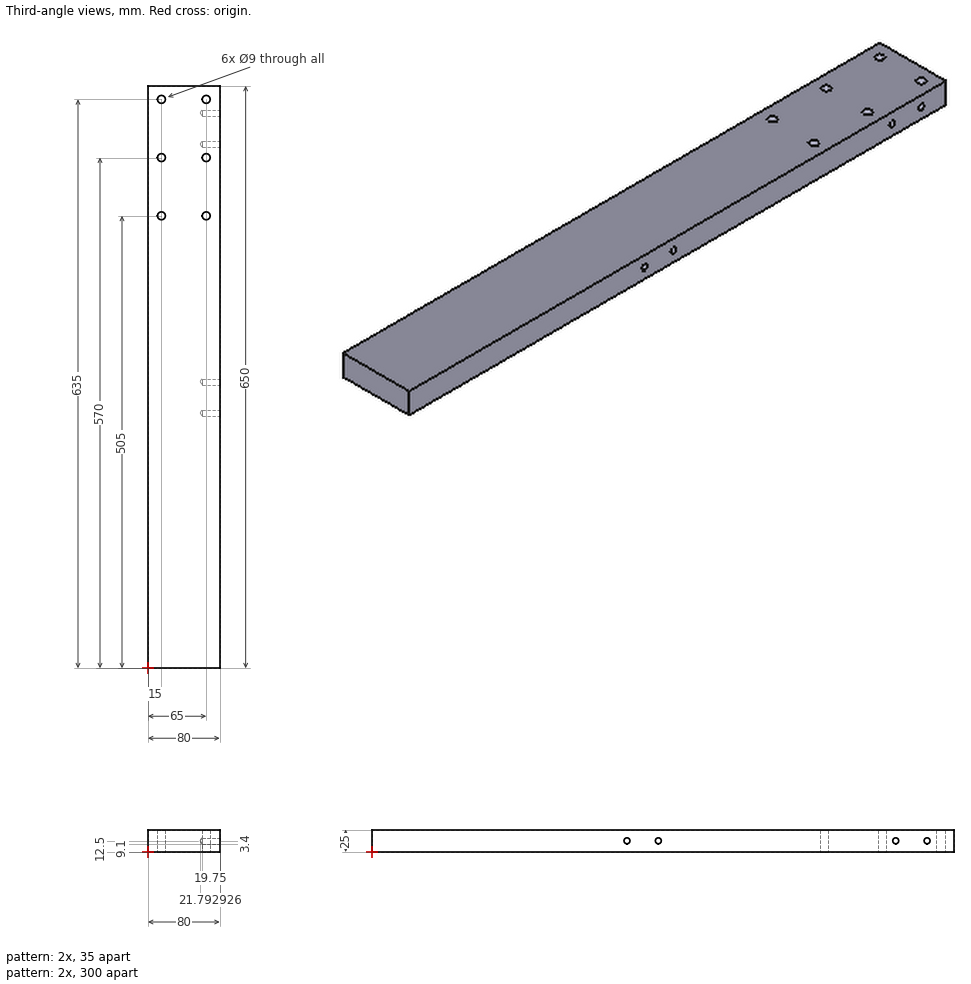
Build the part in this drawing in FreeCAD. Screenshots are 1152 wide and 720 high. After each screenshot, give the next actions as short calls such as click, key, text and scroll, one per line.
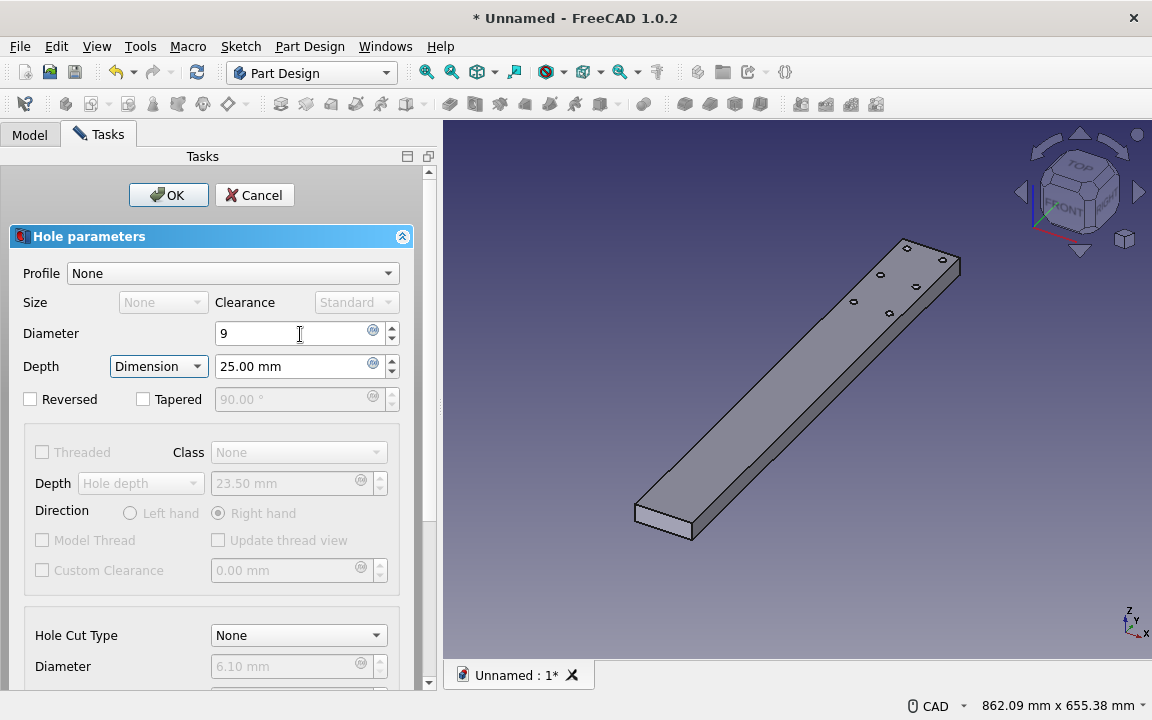
click(160, 366)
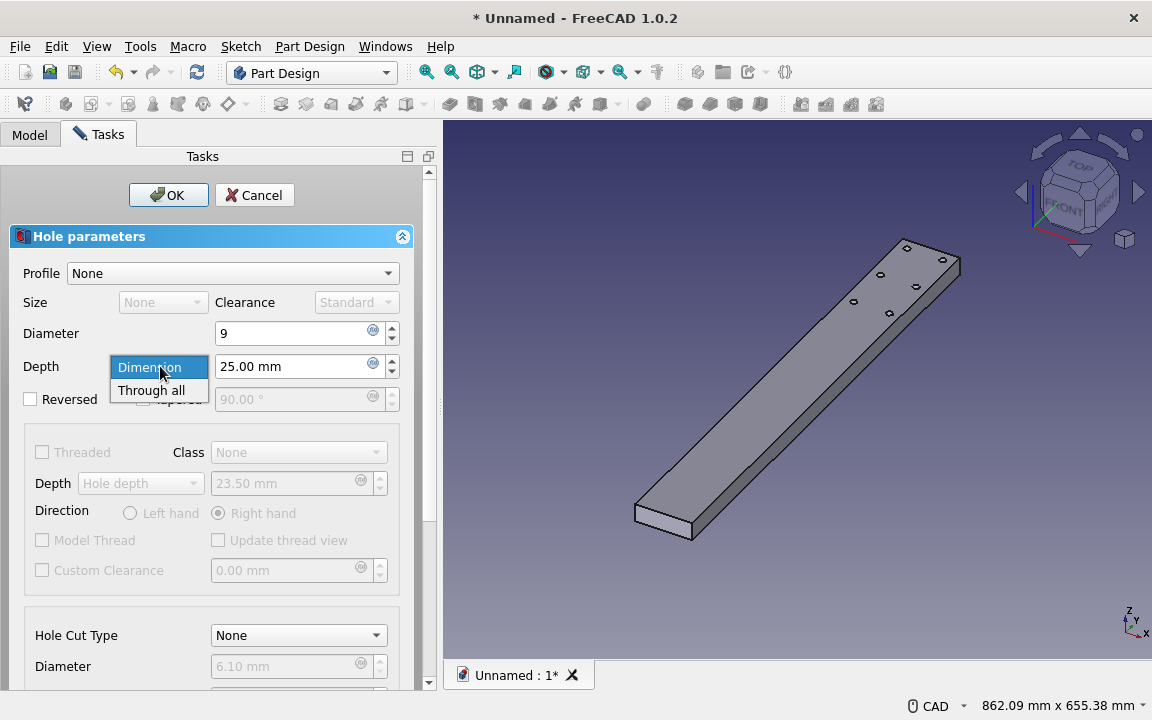
click(158, 390)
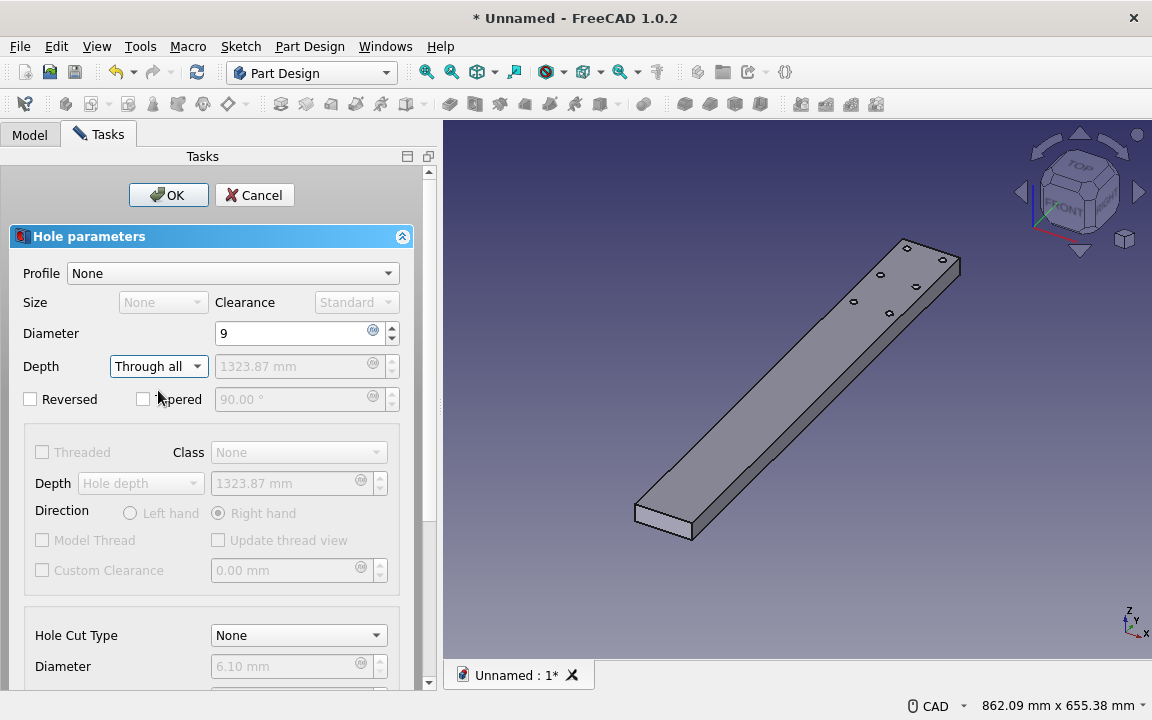
click(169, 195)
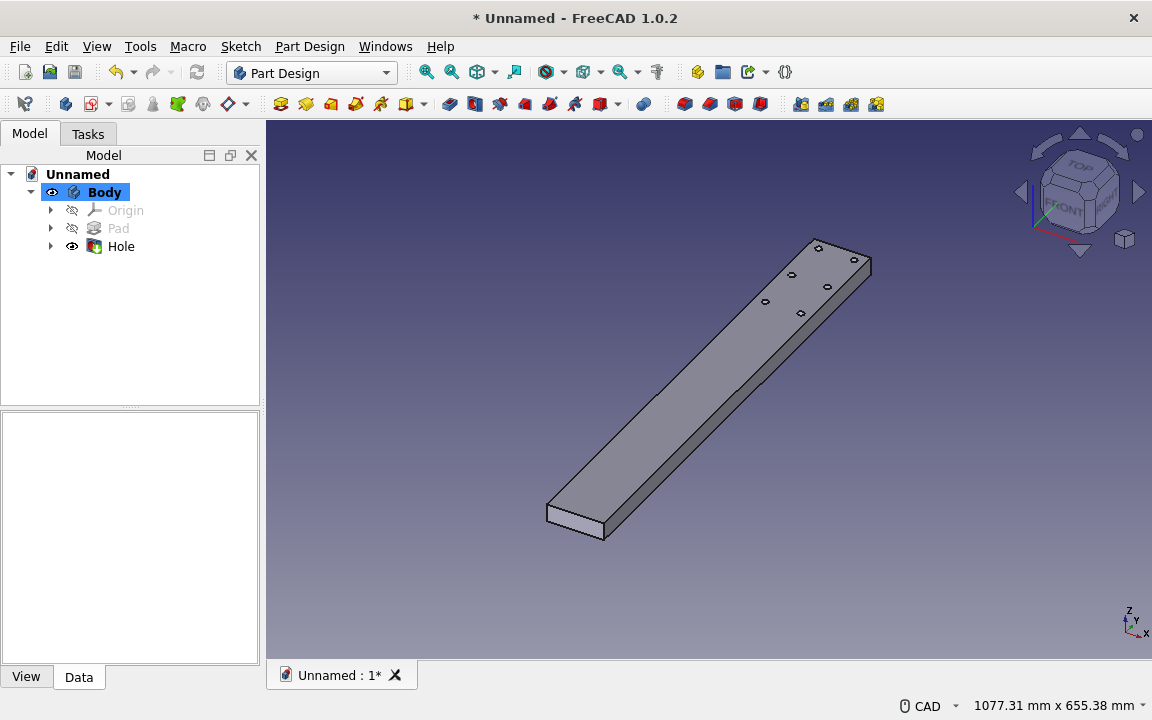
click(51, 210)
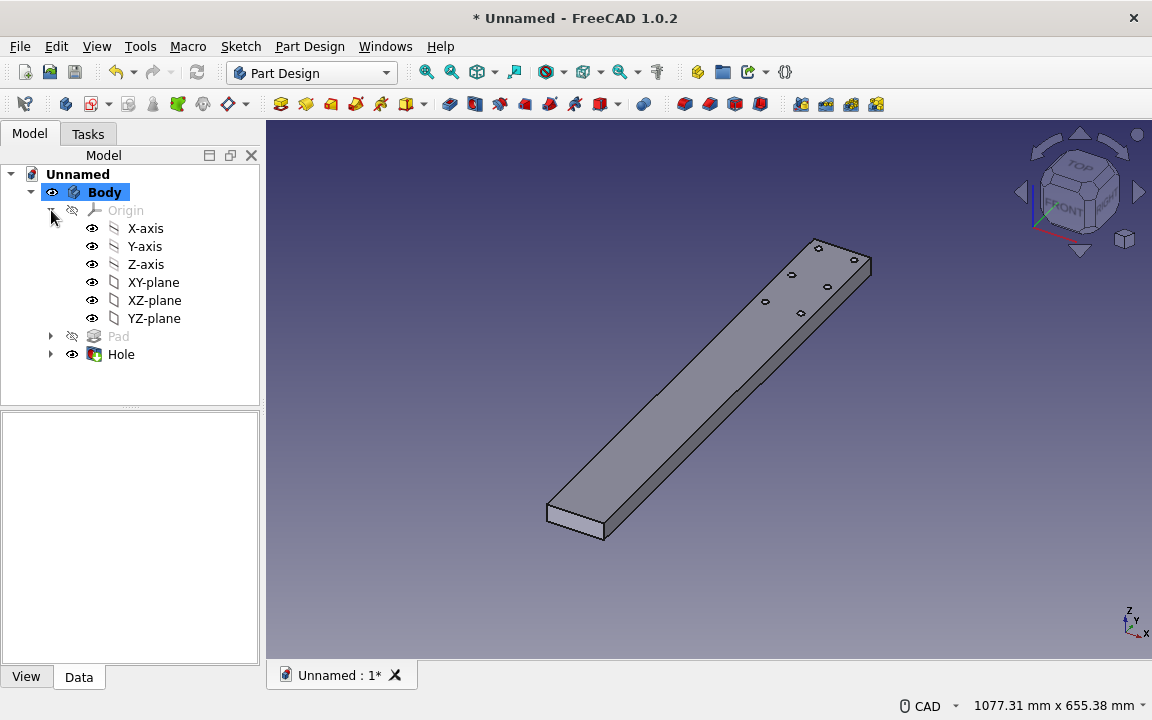
click(137, 300)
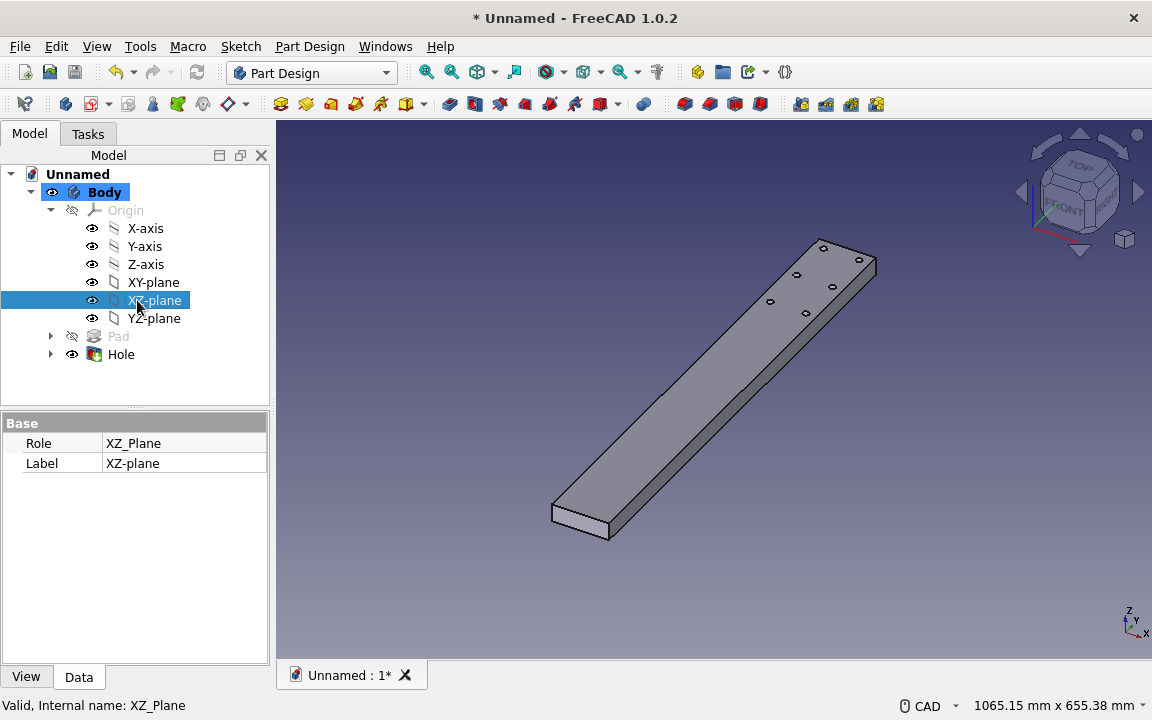
click(228, 104)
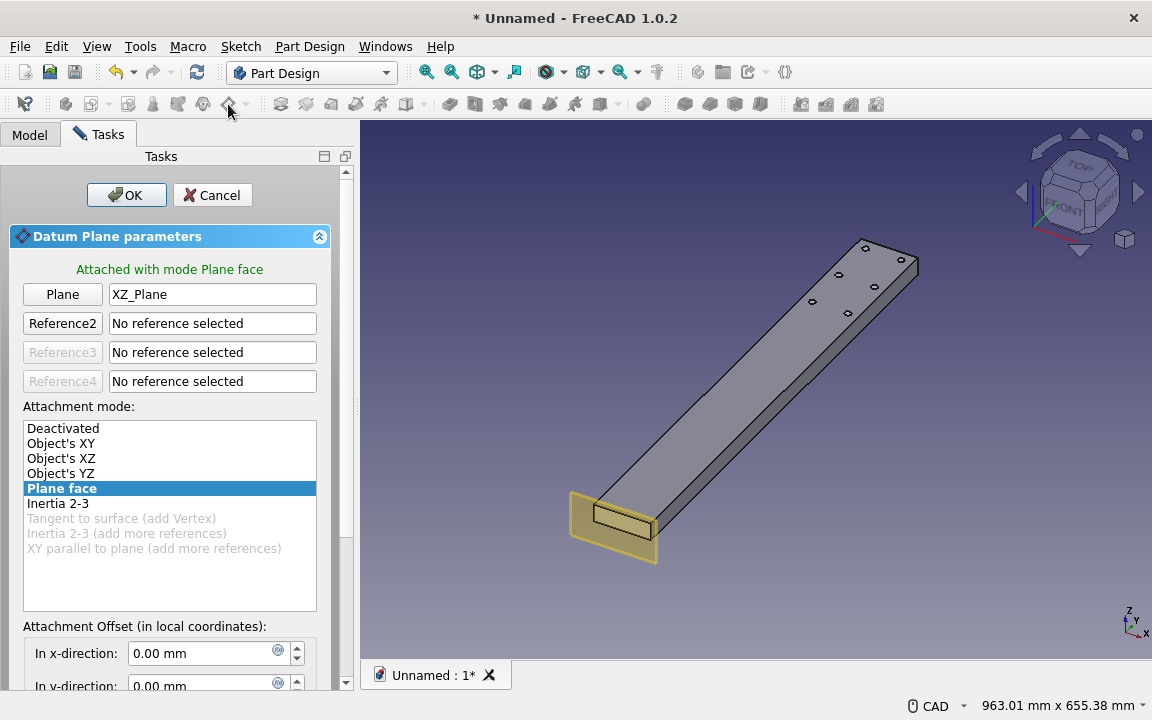
scroll(346, 428, down, 2)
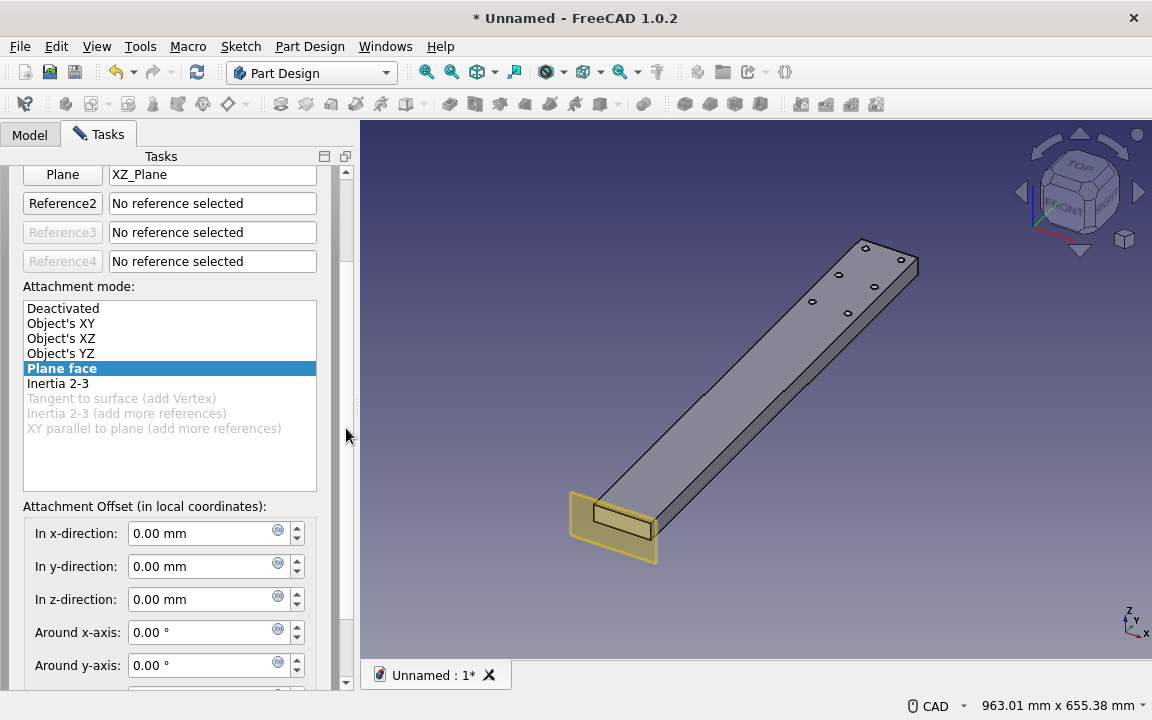
triple_click(210, 600)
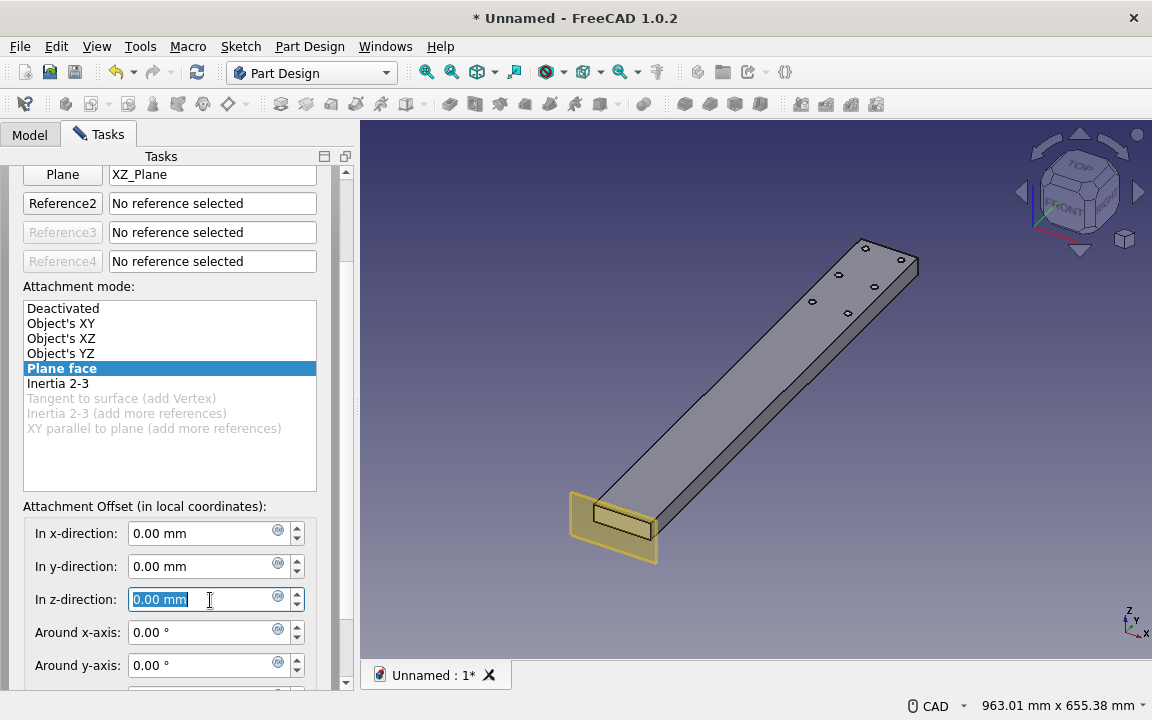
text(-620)
key(Tab)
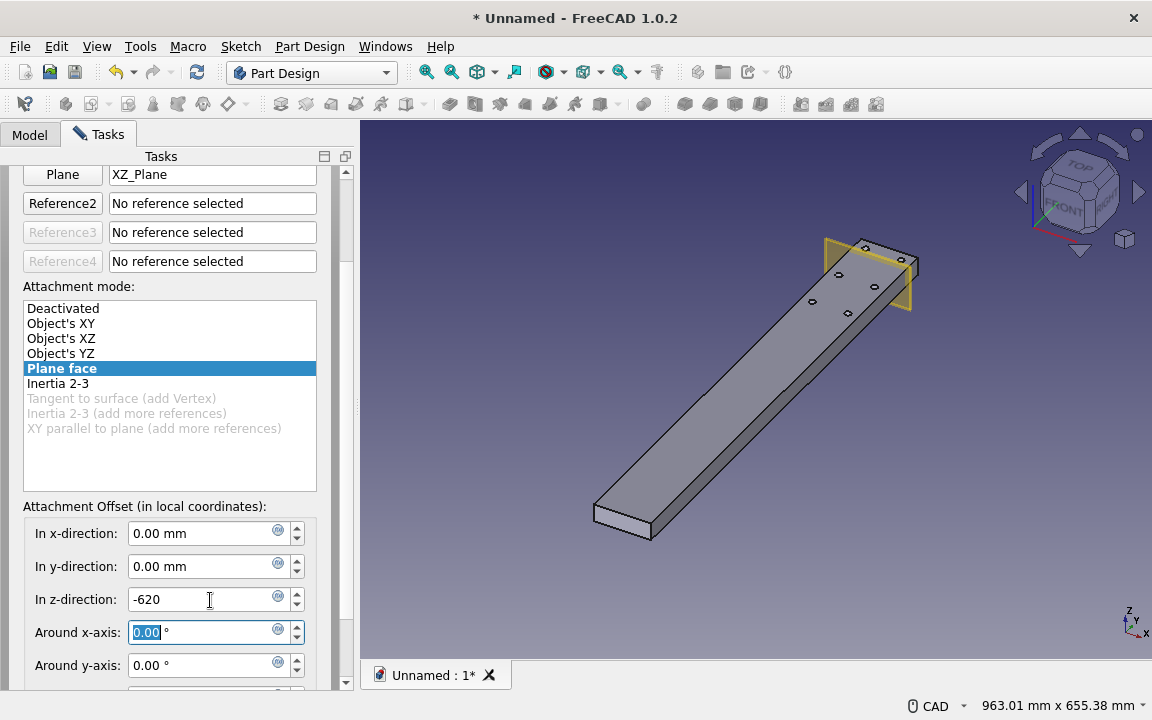
scroll(346, 428, up, 3)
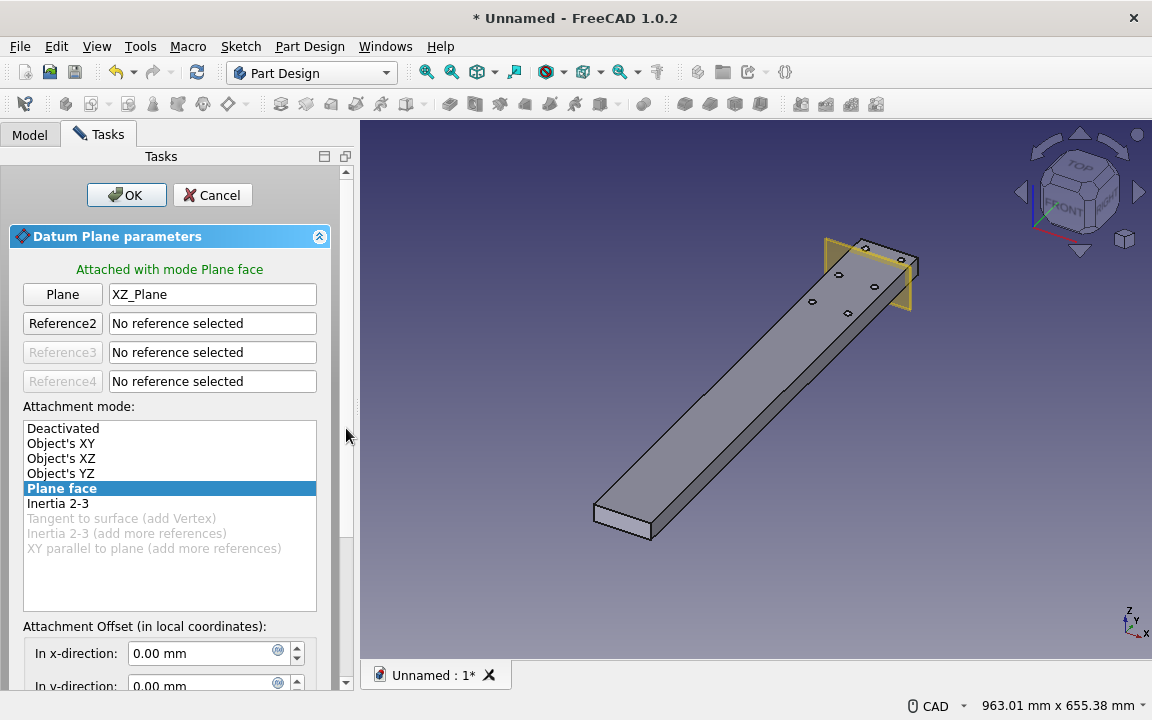
click(127, 195)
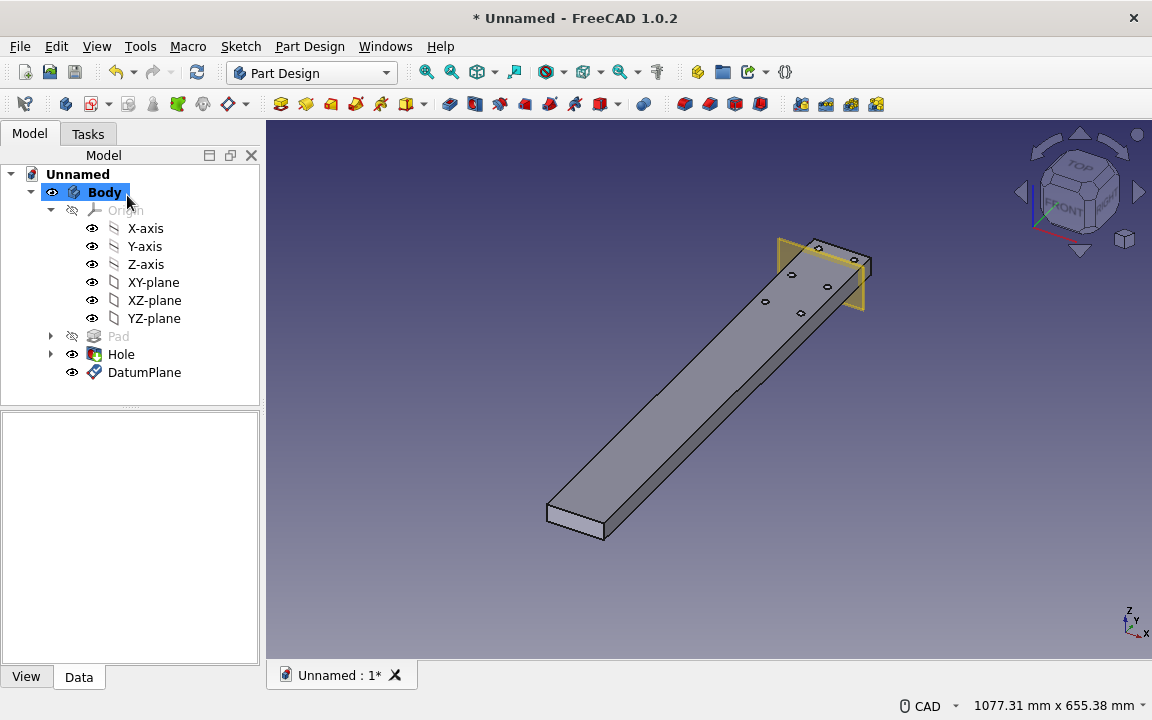
click(117, 372)